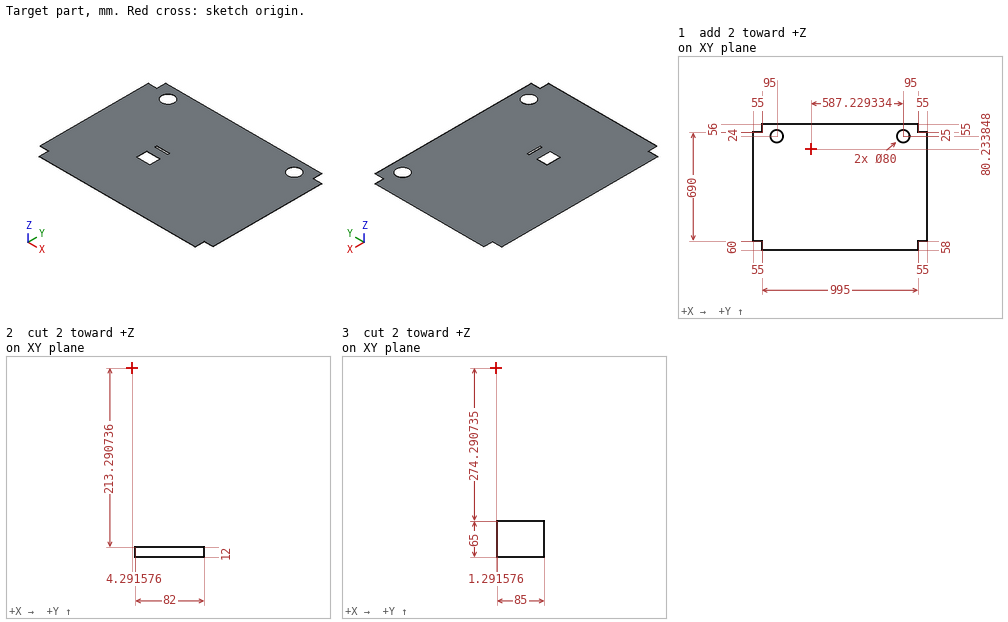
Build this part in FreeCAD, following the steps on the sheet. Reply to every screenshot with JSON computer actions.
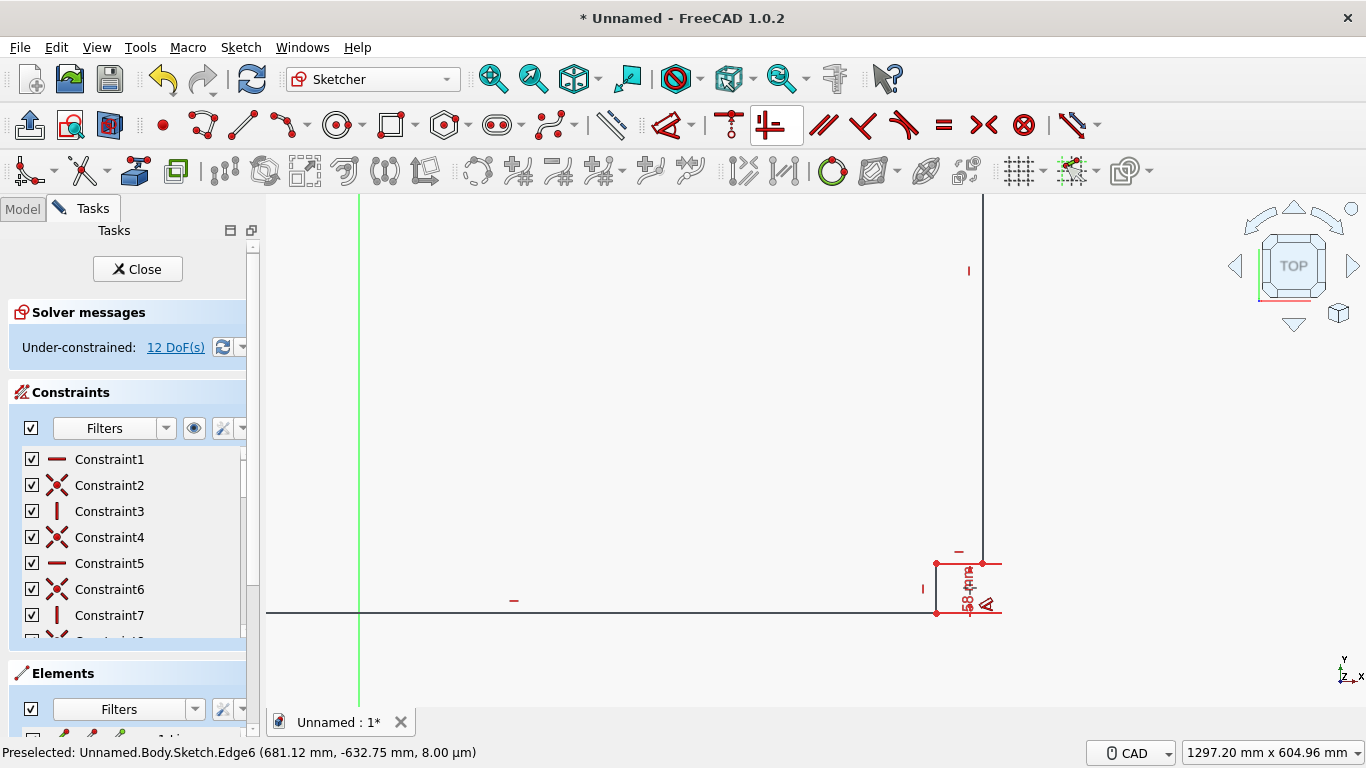
{"action": "left_click", "coordinate": [950, 564]}
{"action": "left_click", "coordinate": [959, 530]}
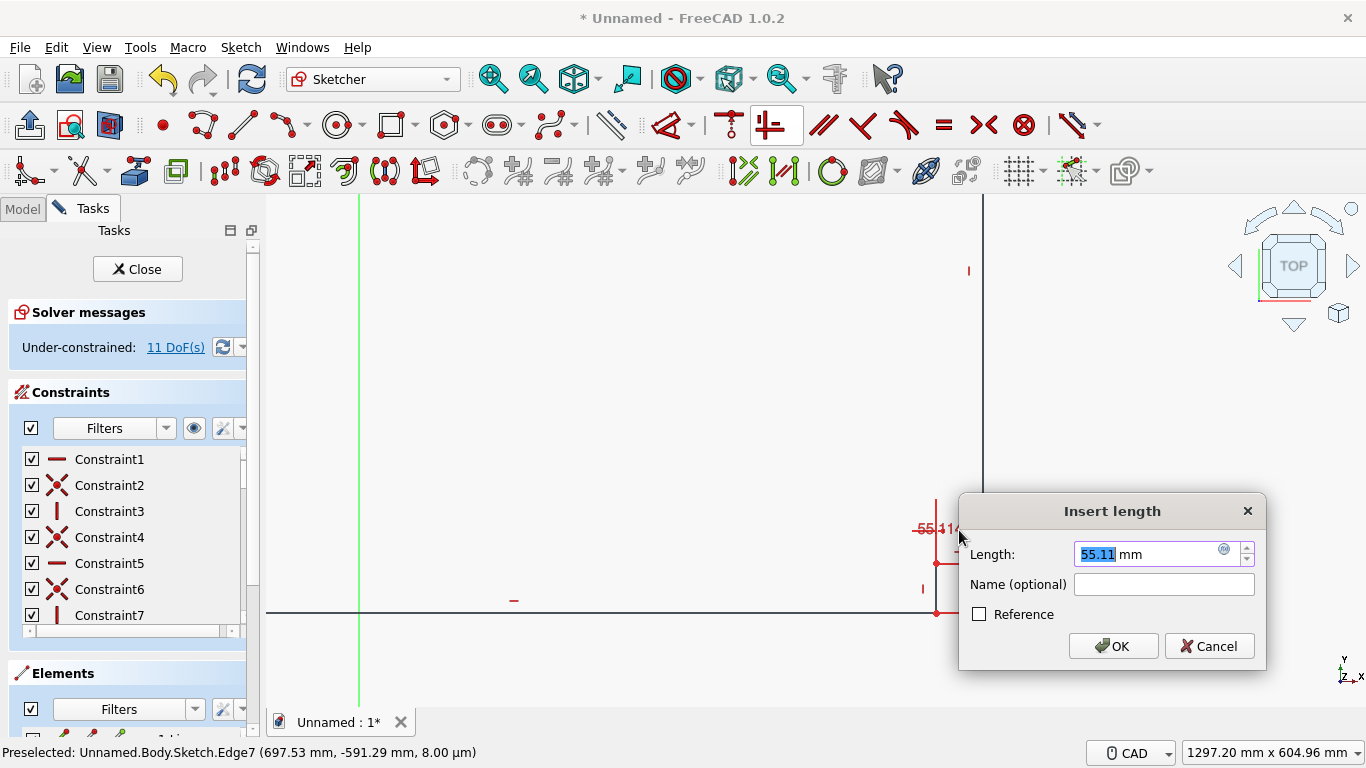
{"action": "type", "text": "55"}
{"action": "key", "text": "Return"}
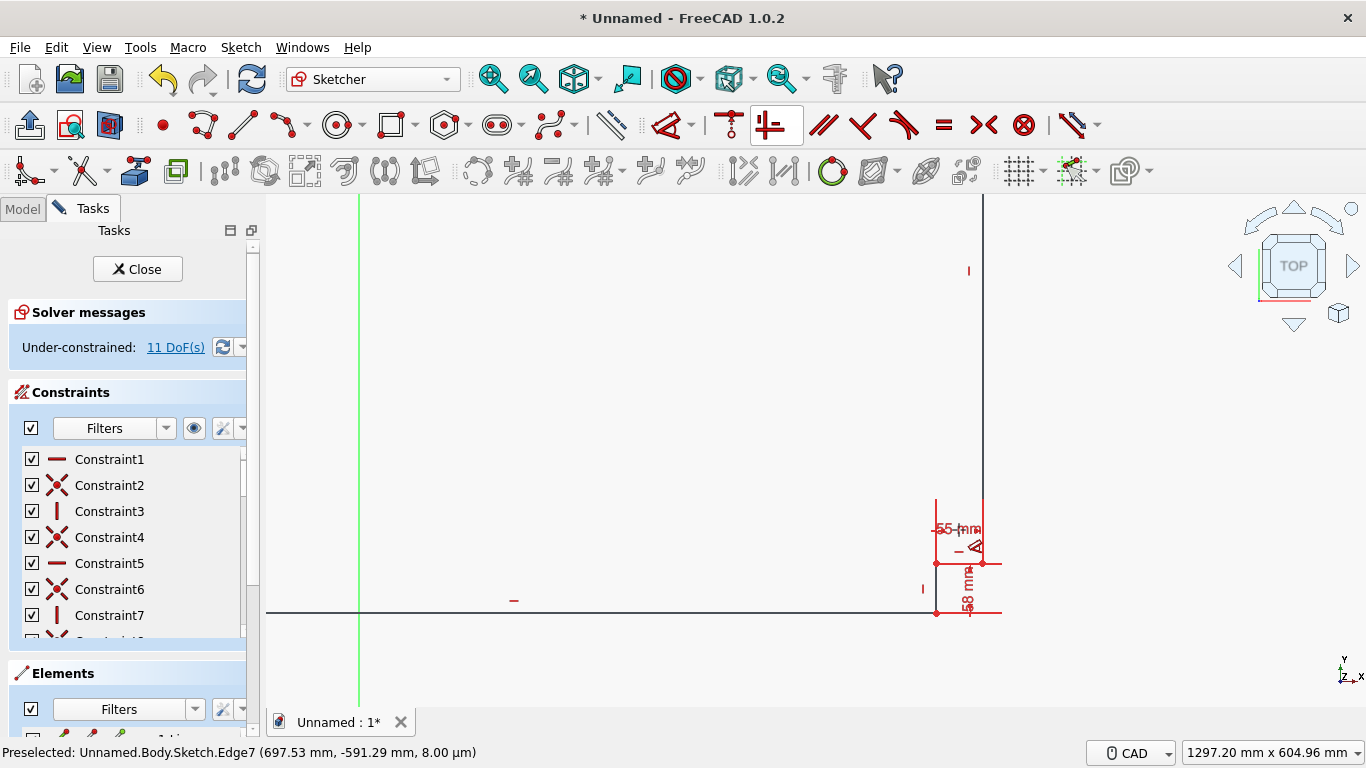
{"action": "scroll", "coordinate": [937, 599], "scroll_direction": "down", "scroll_amount": 4}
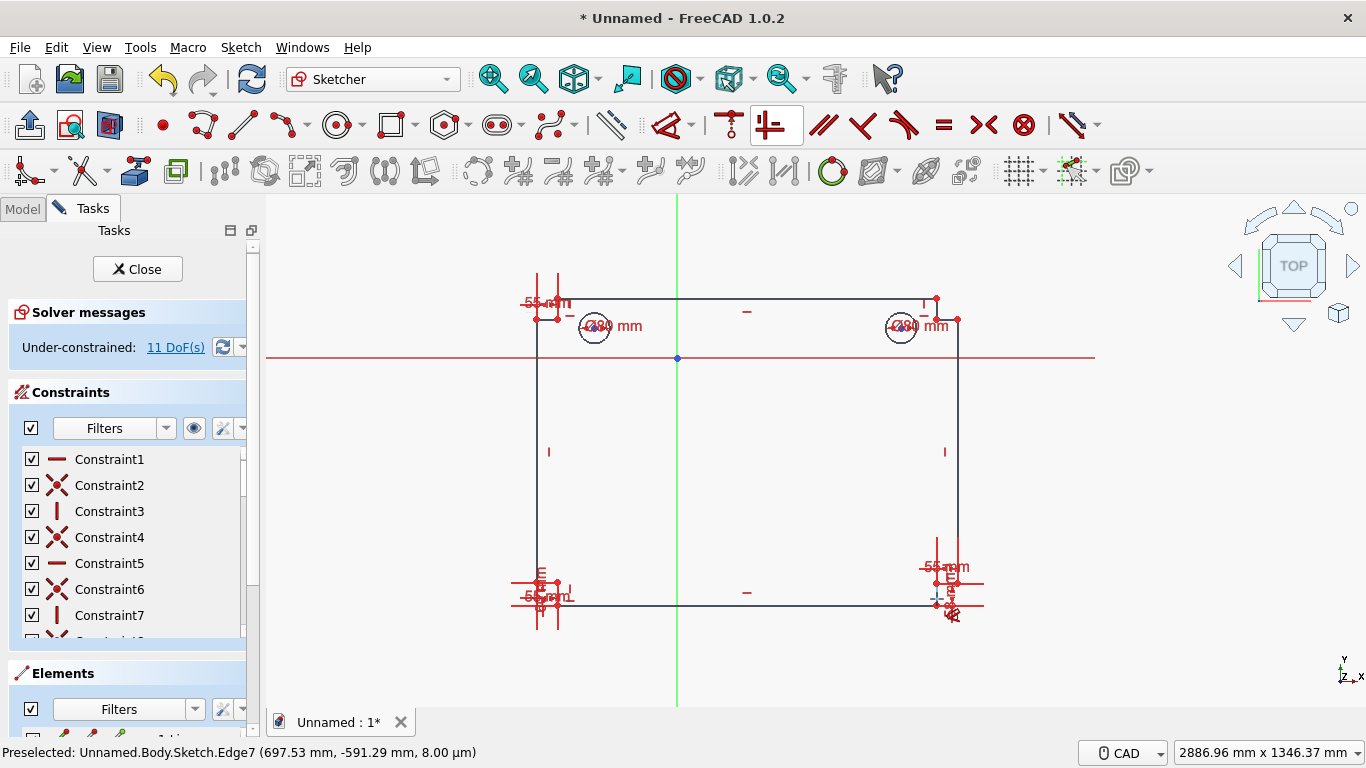
{"action": "scroll", "coordinate": [952, 320], "scroll_direction": "up", "scroll_amount": 4}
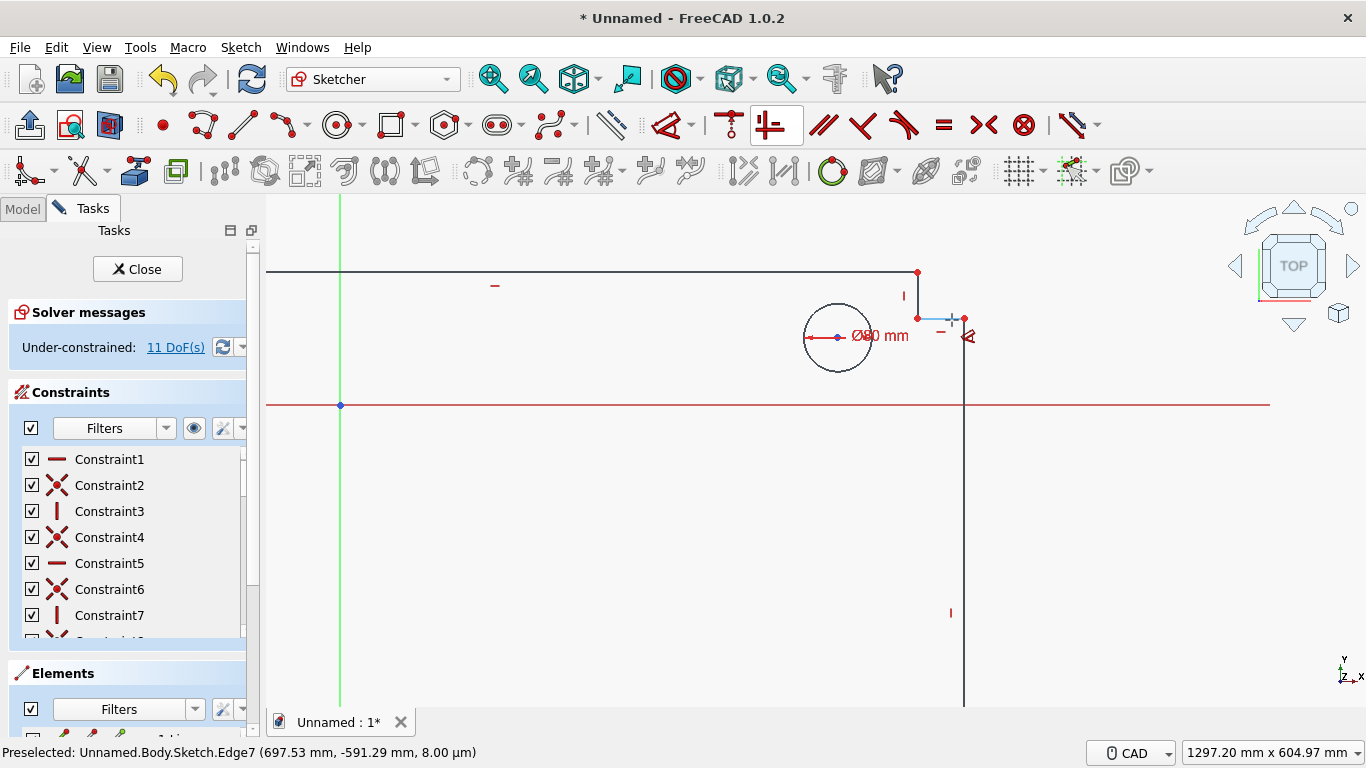
{"action": "left_click", "coordinate": [950, 319]}
{"action": "left_click", "coordinate": [941, 285]}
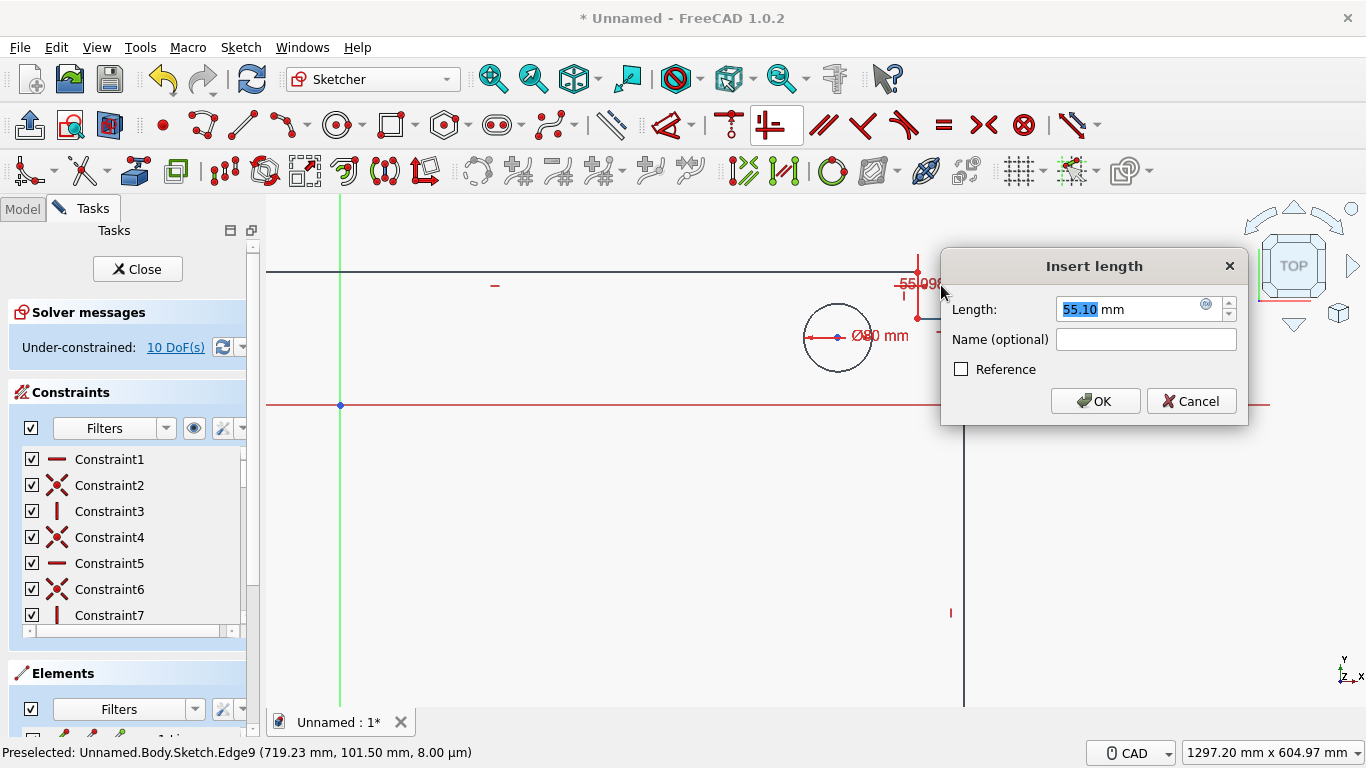
{"action": "type", "text": "55"}
{"action": "key", "text": "Return"}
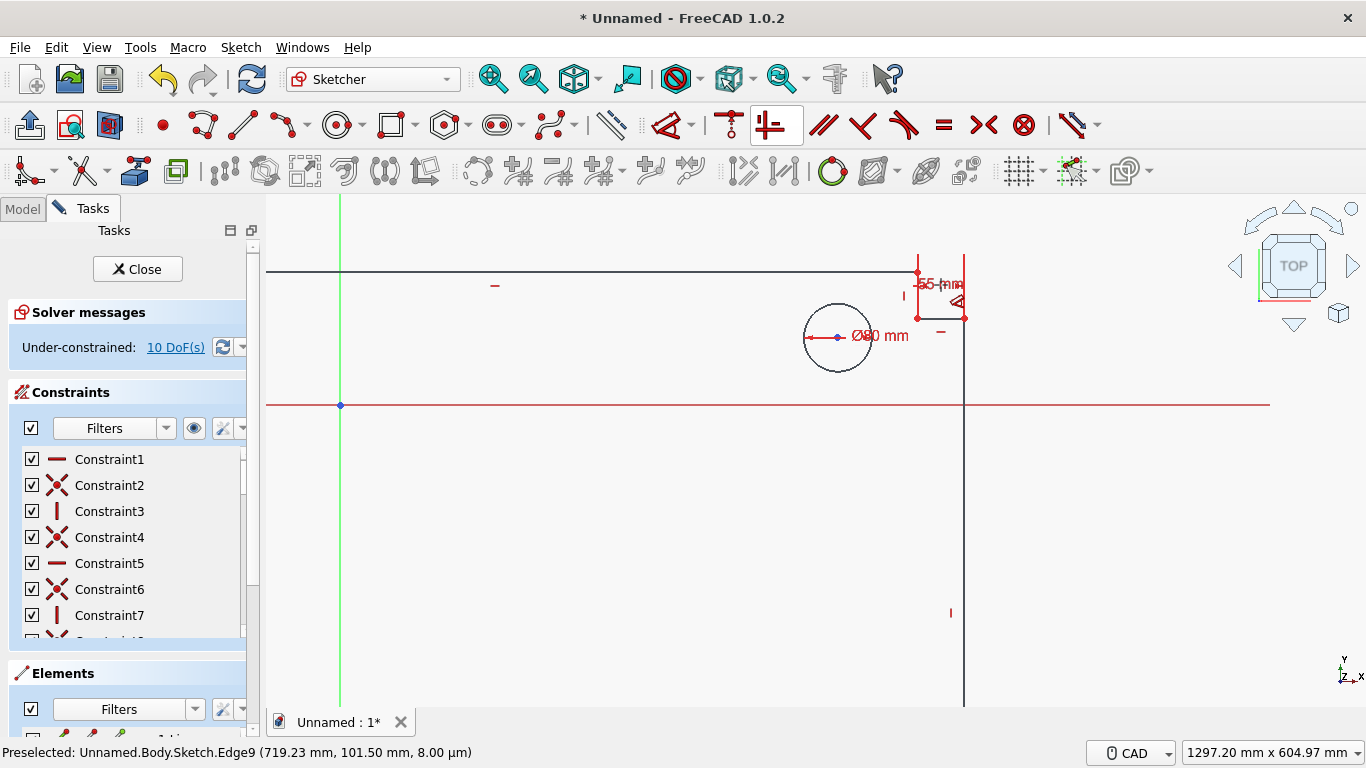
{"action": "left_click", "coordinate": [918, 305]}
{"action": "left_click", "coordinate": [884, 306]}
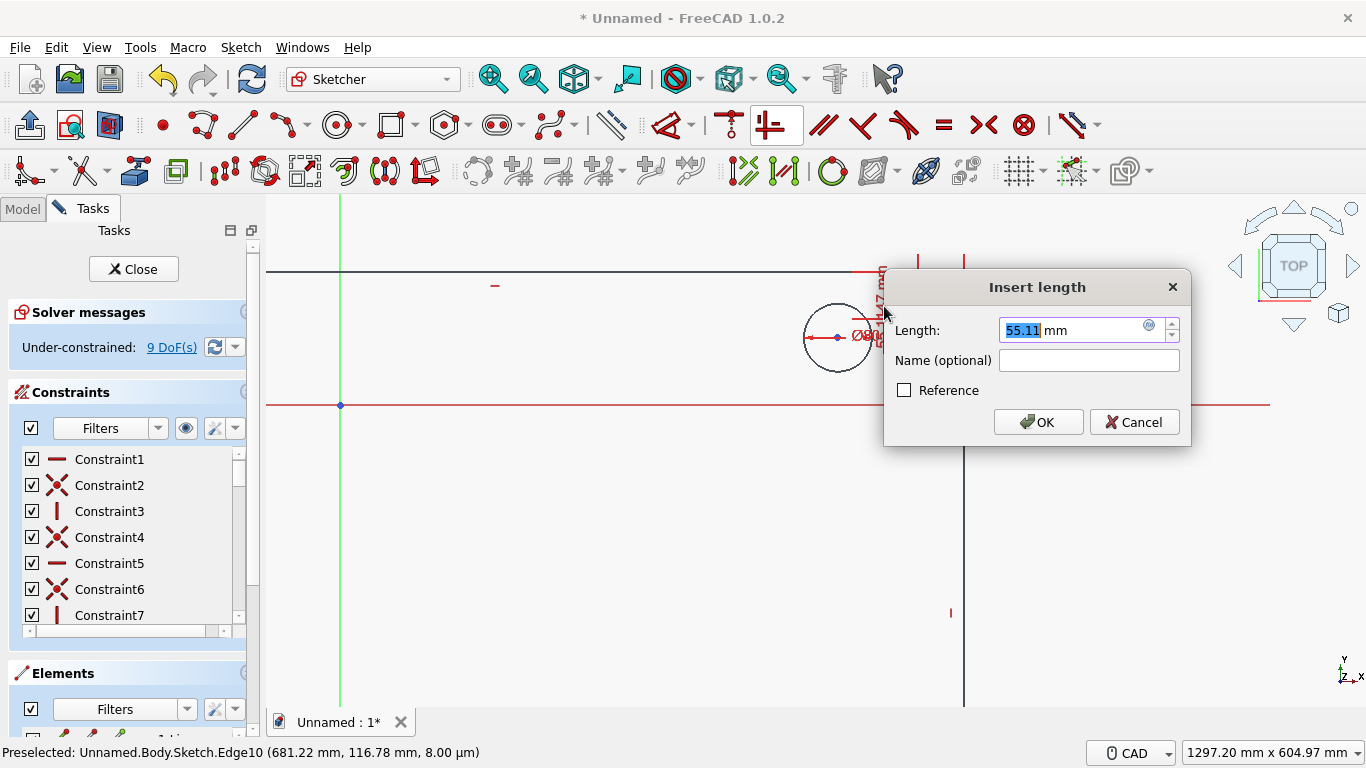
{"action": "type", "text": "55"}
{"action": "key", "text": "Return"}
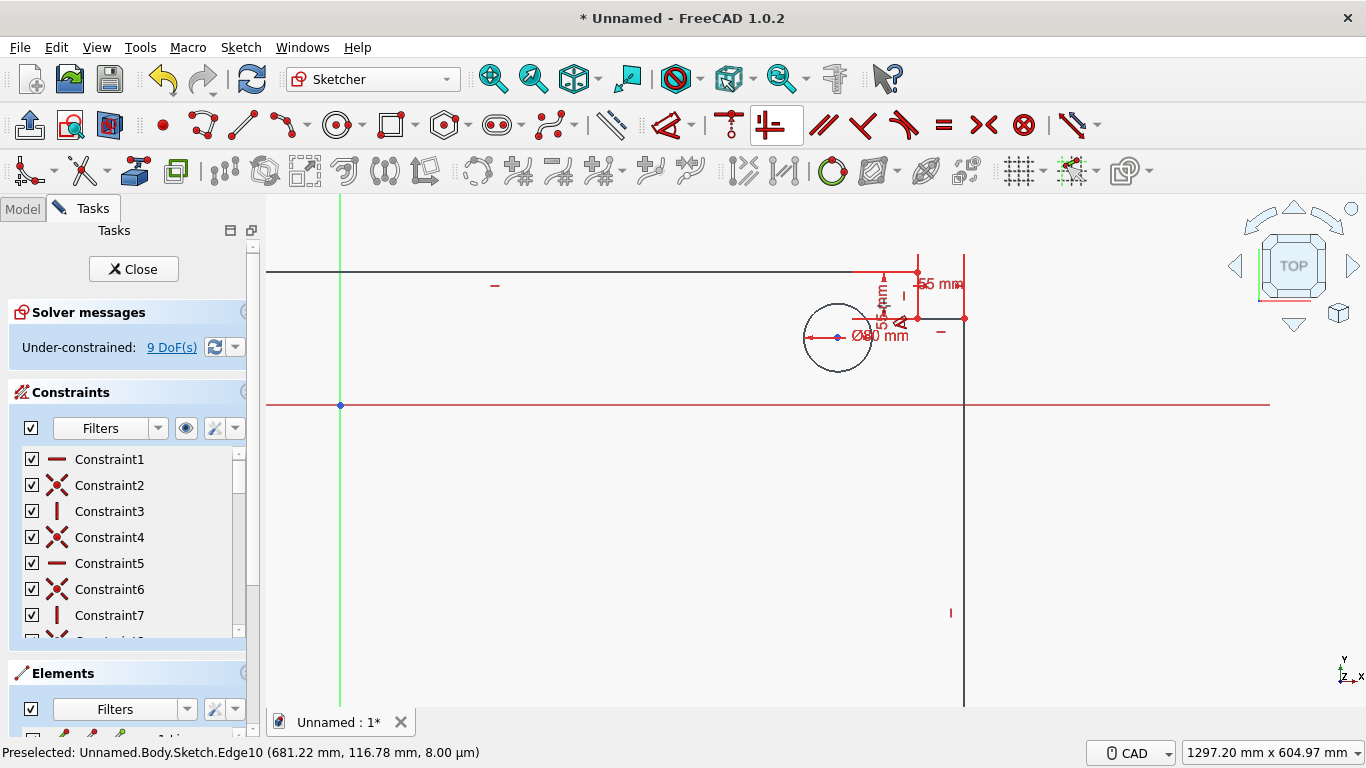
{"action": "scroll", "coordinate": [952, 320], "scroll_direction": "down", "scroll_amount": 4}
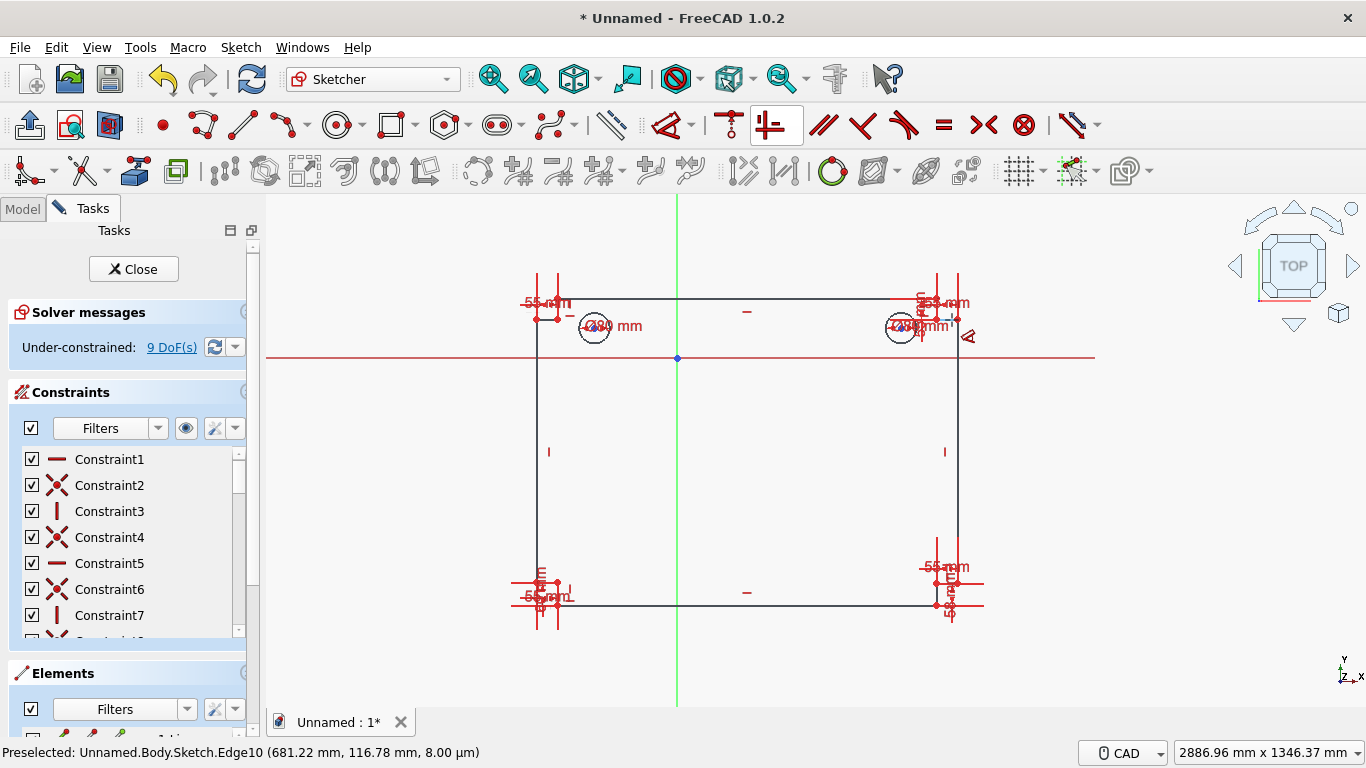
{"action": "scroll", "coordinate": [558, 305], "scroll_direction": "up", "scroll_amount": 4}